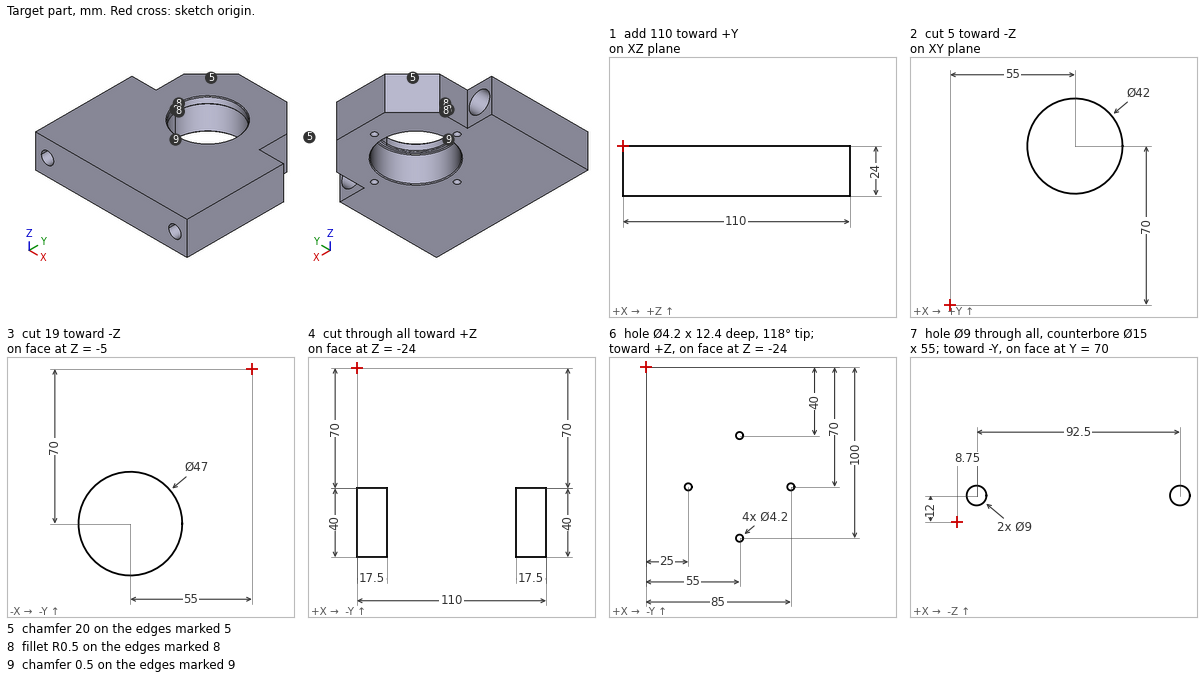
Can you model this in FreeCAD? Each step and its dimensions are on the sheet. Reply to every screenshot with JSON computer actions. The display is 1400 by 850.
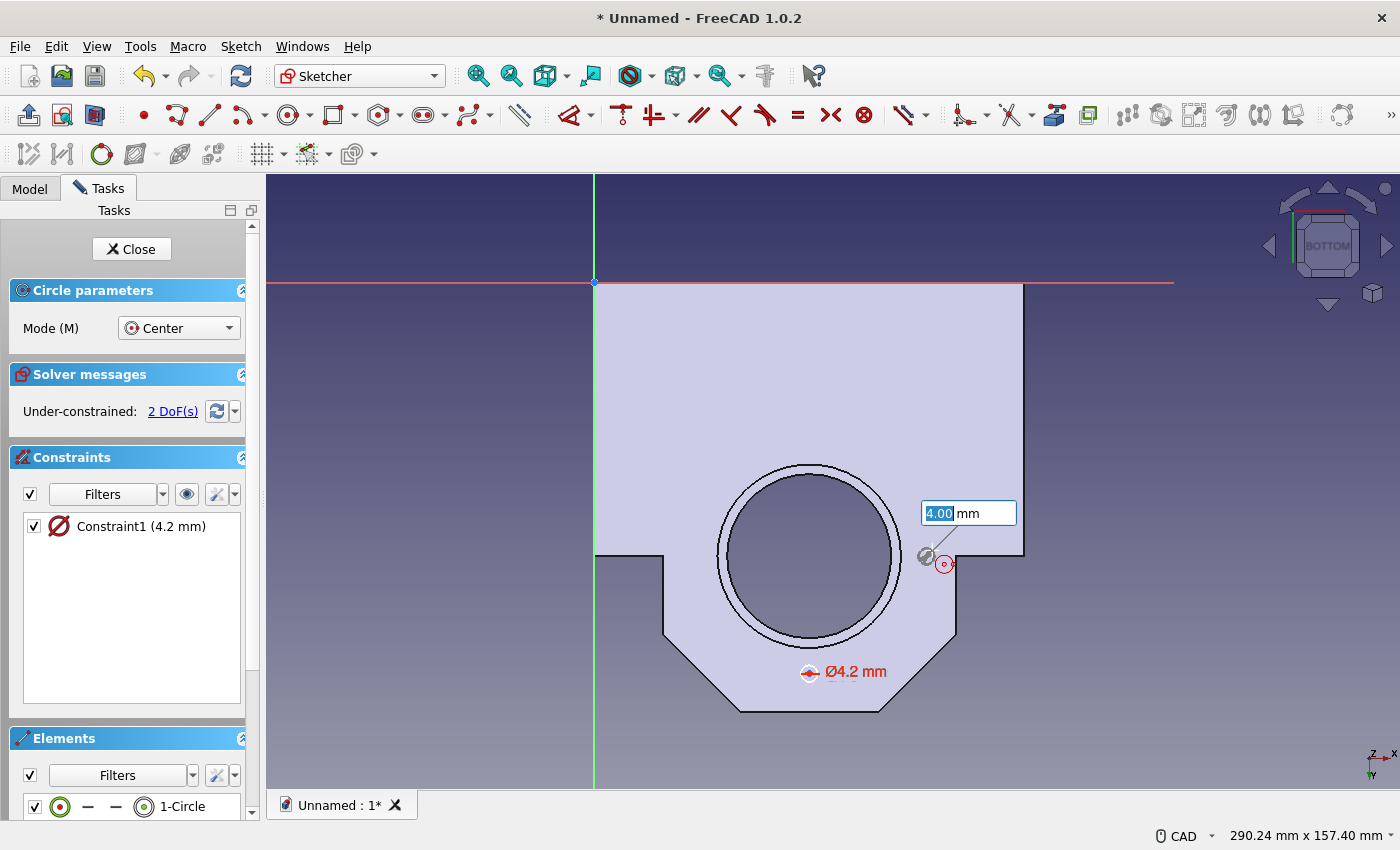
{"action": "type", "text": "4.2"}
{"action": "key", "text": "Return"}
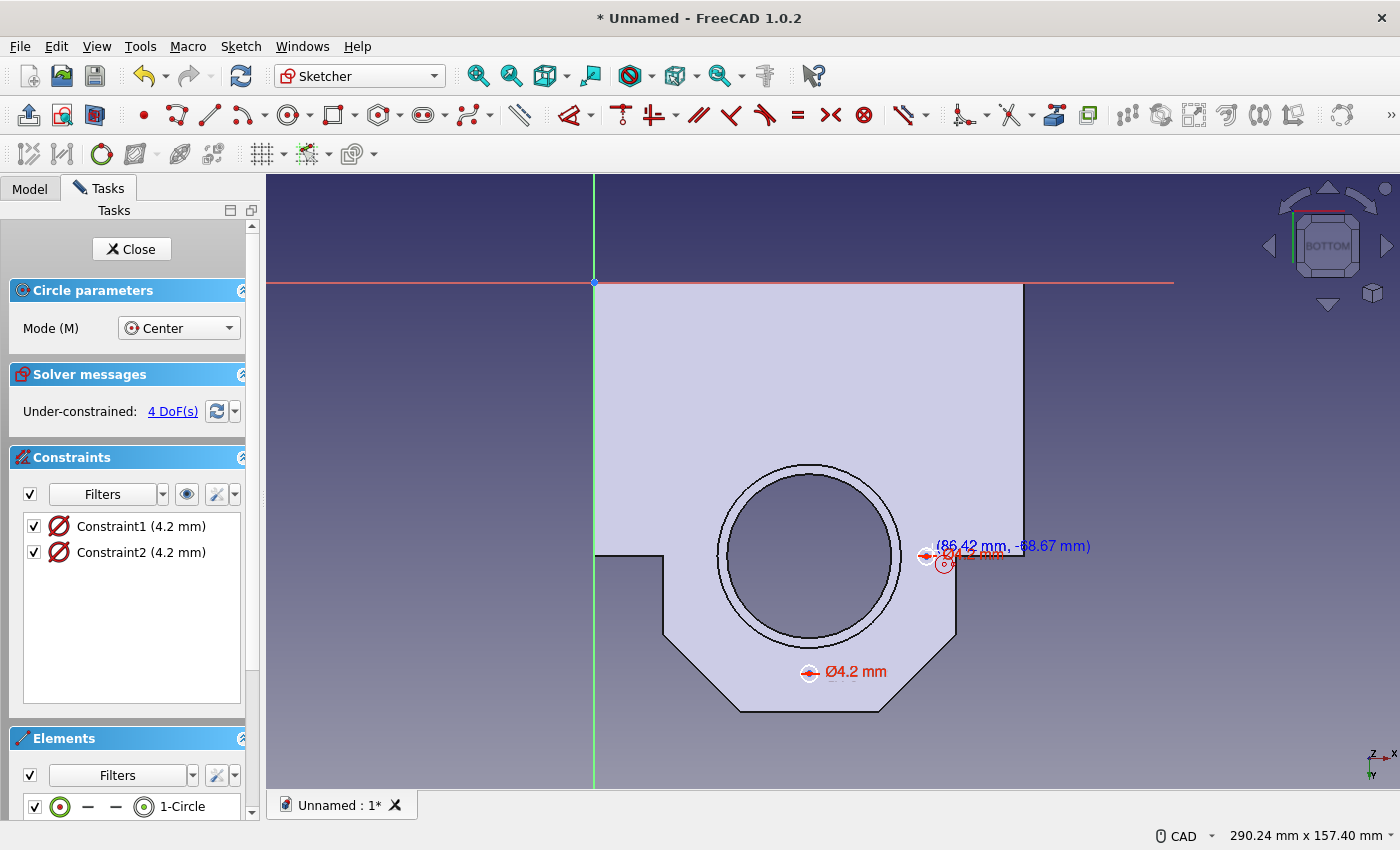
{"action": "scroll", "coordinate": [809, 439], "scroll_direction": "up", "scroll_amount": 6}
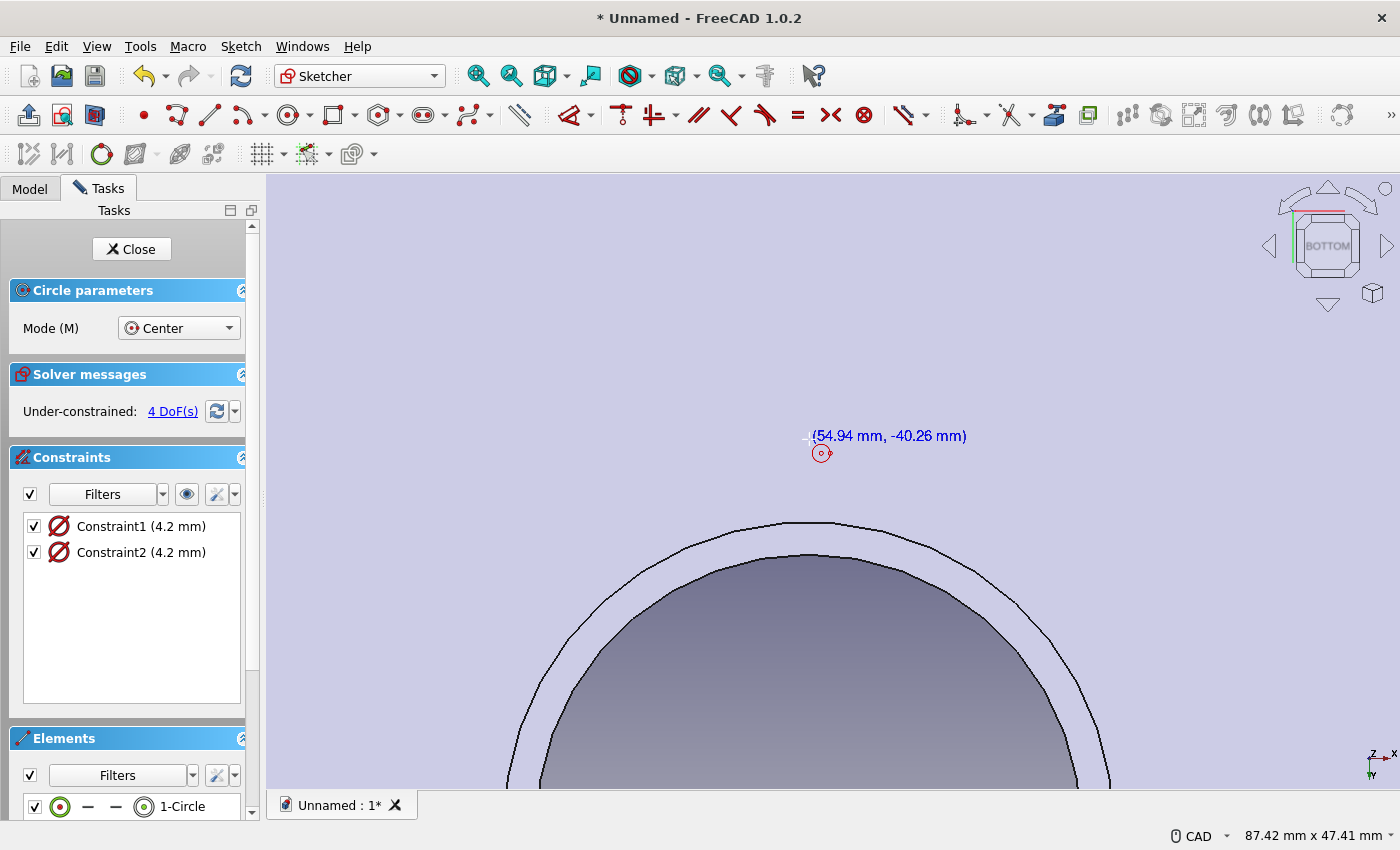
{"action": "left_click", "coordinate": [809, 438]}
{"action": "mouse_move", "coordinate": [828, 419]}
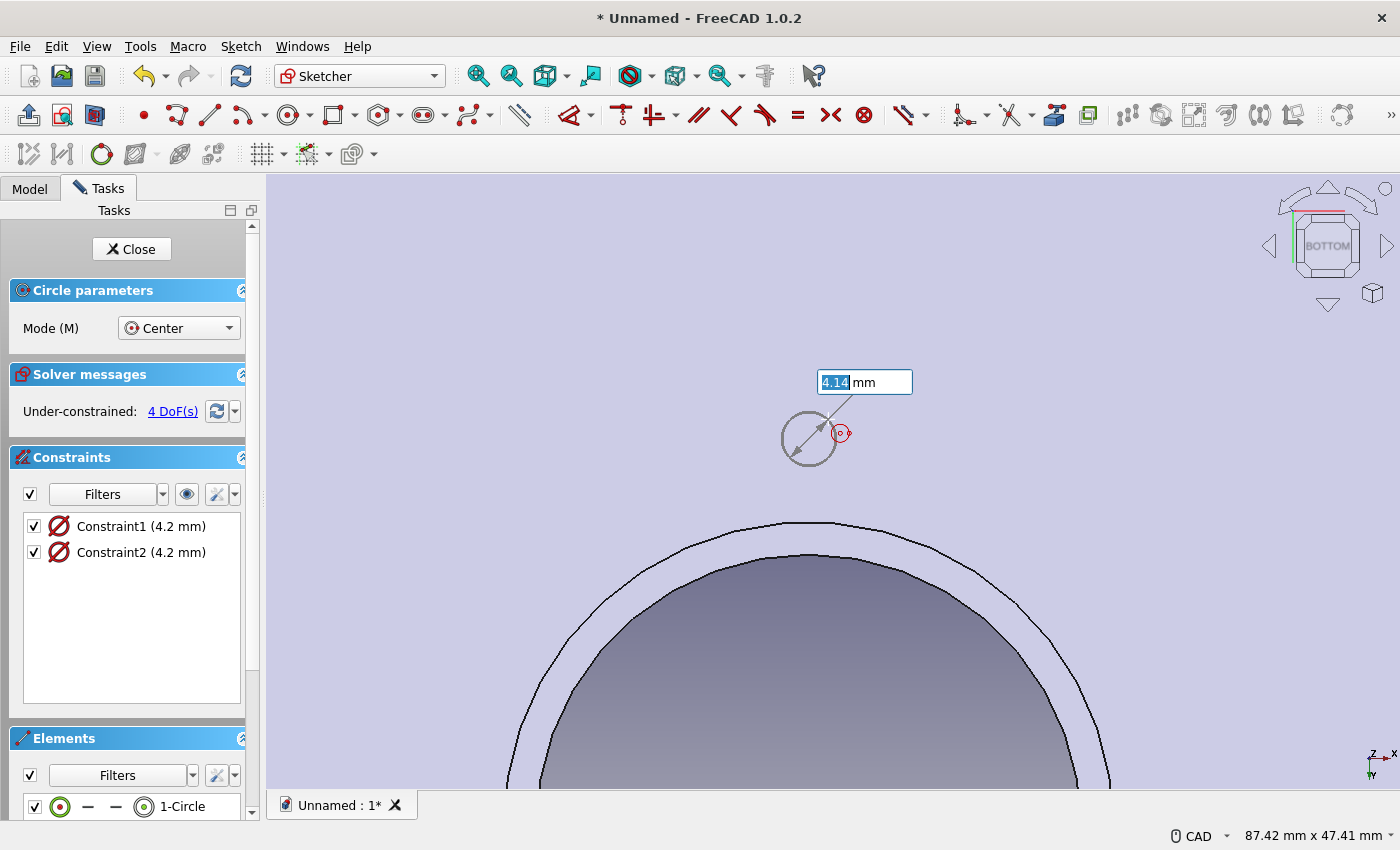
{"action": "type", "text": "4.2"}
{"action": "key", "text": "Return"}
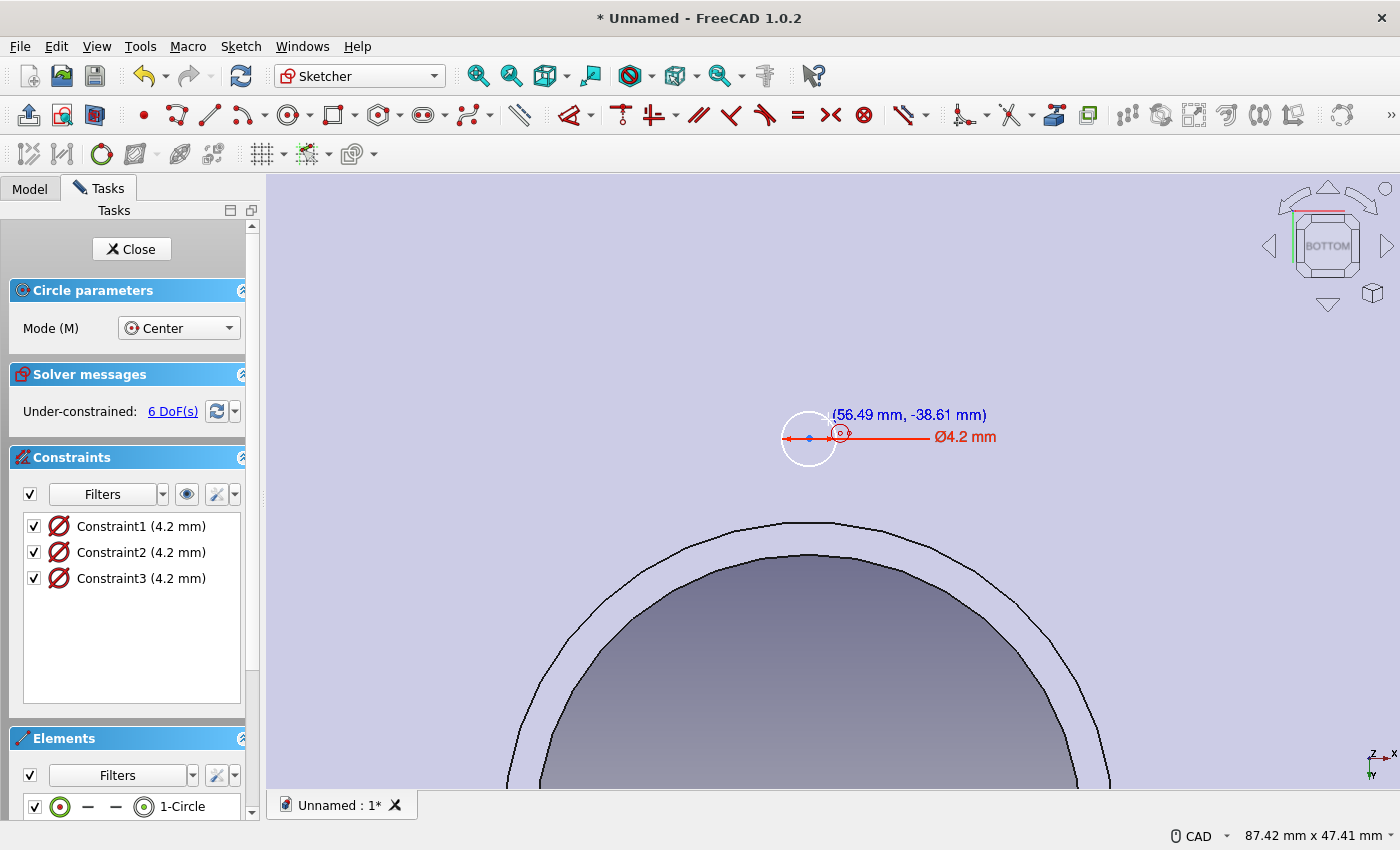
{"action": "scroll", "coordinate": [810, 438], "scroll_direction": "down", "scroll_amount": 6}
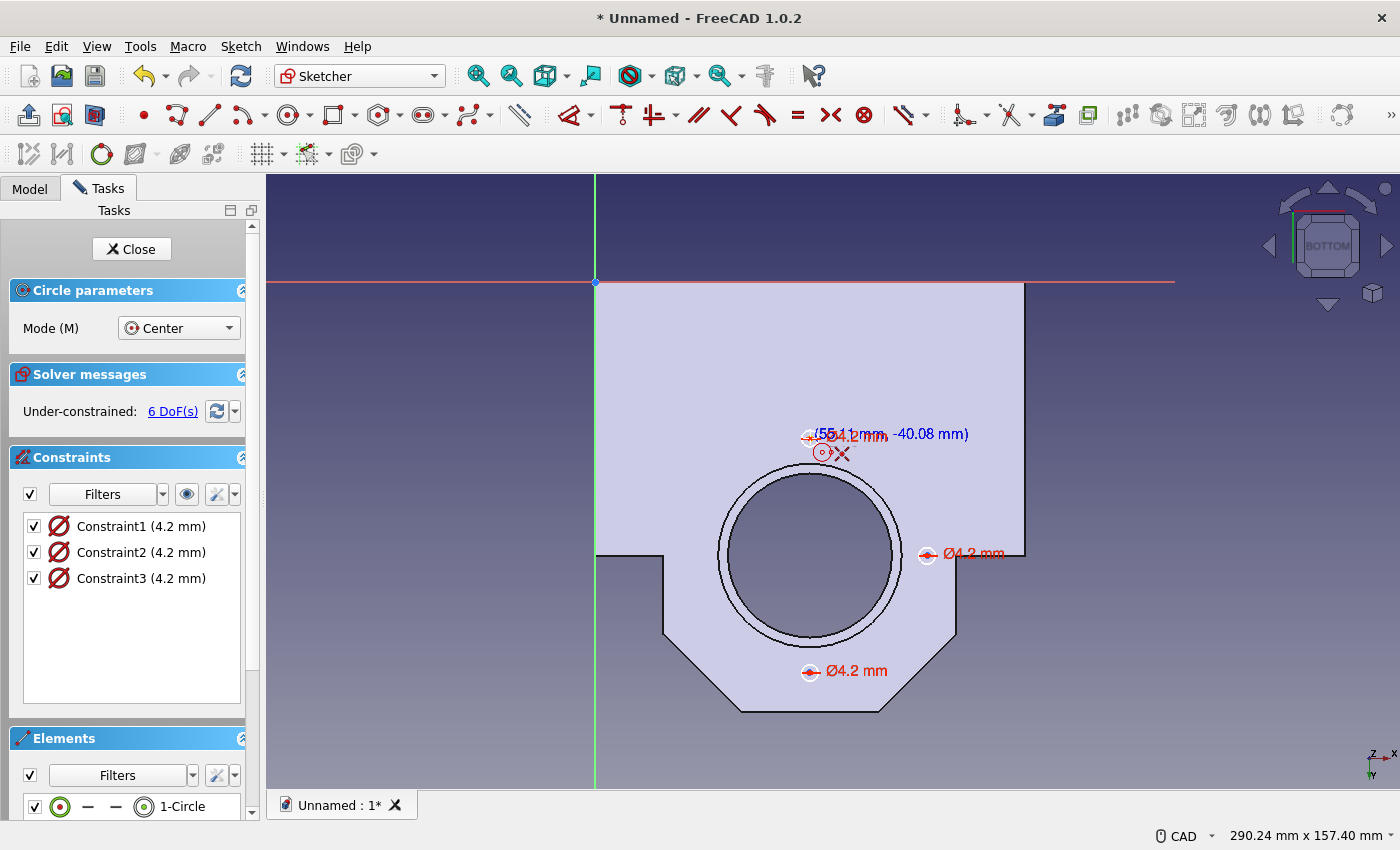
{"action": "scroll", "coordinate": [693, 556], "scroll_direction": "up", "scroll_amount": 6}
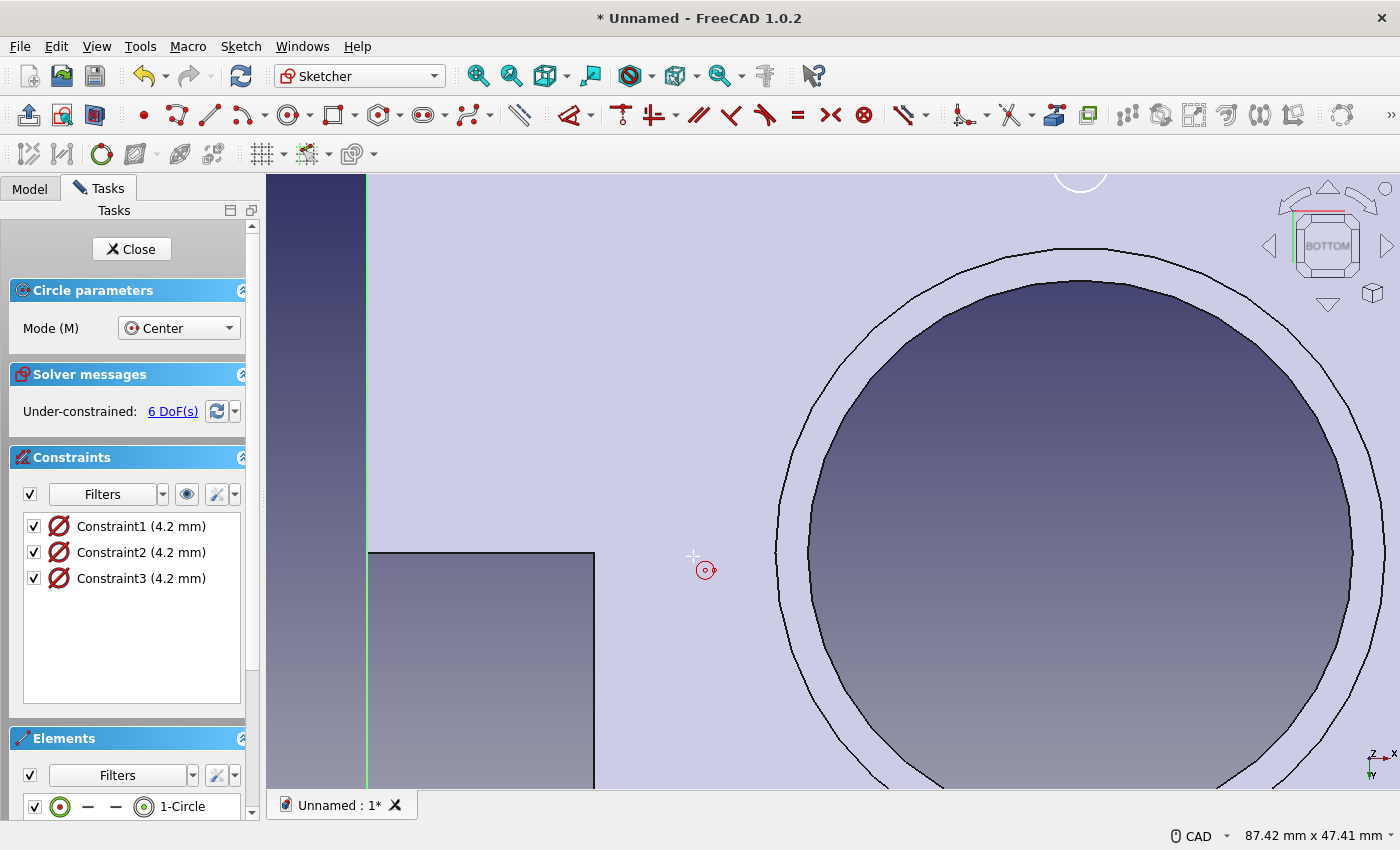
{"action": "left_click", "coordinate": [691, 553]}
{"action": "mouse_move", "coordinate": [710, 534]}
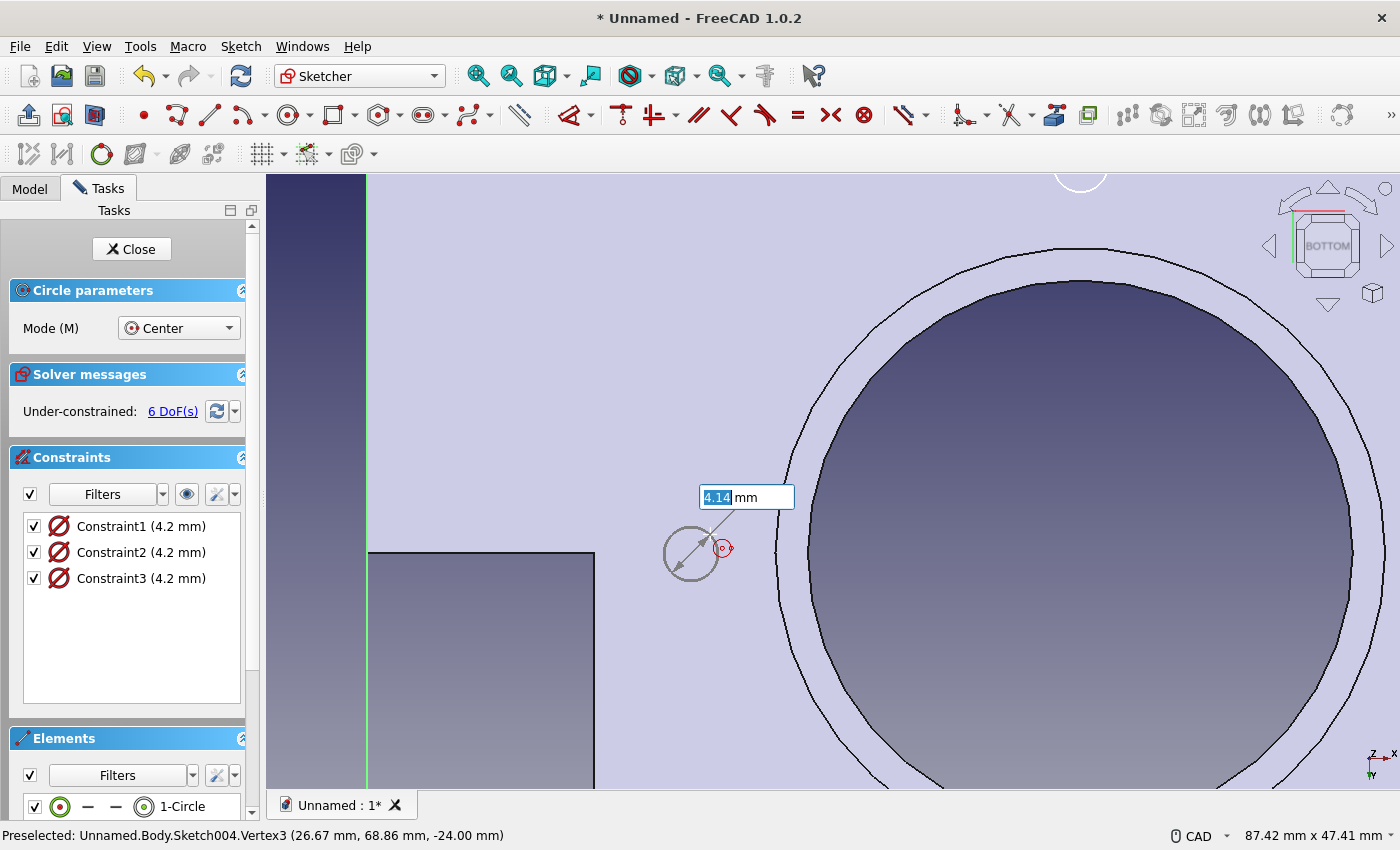
{"action": "type", "text": "4.2"}
{"action": "key", "text": "Return"}
{"action": "key", "text": "Escape"}